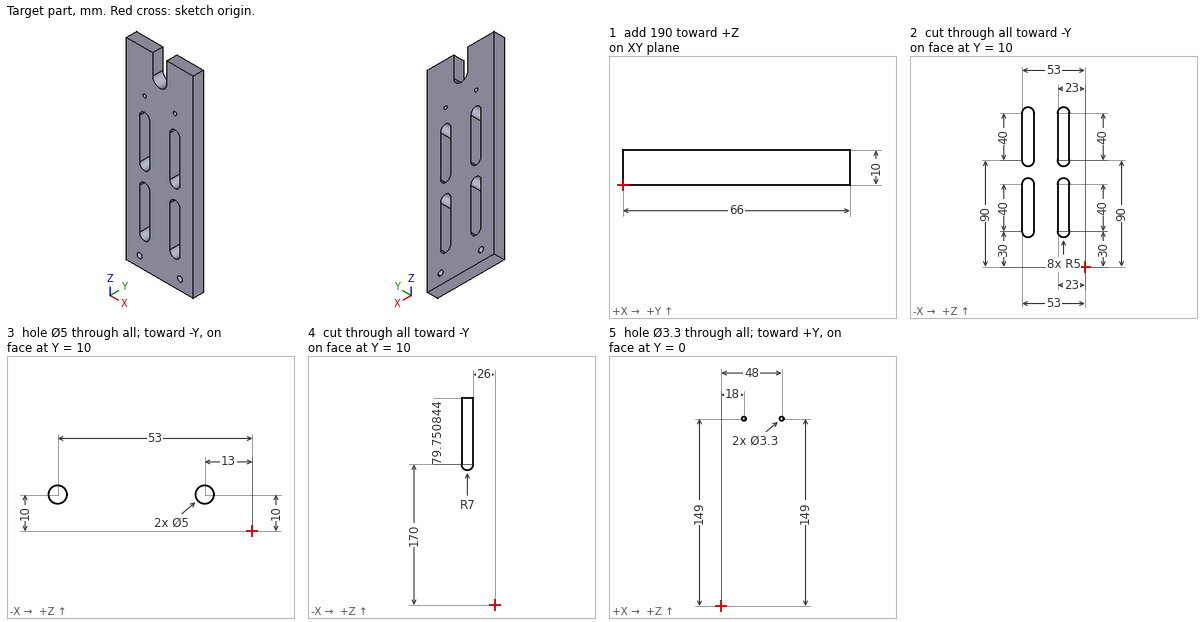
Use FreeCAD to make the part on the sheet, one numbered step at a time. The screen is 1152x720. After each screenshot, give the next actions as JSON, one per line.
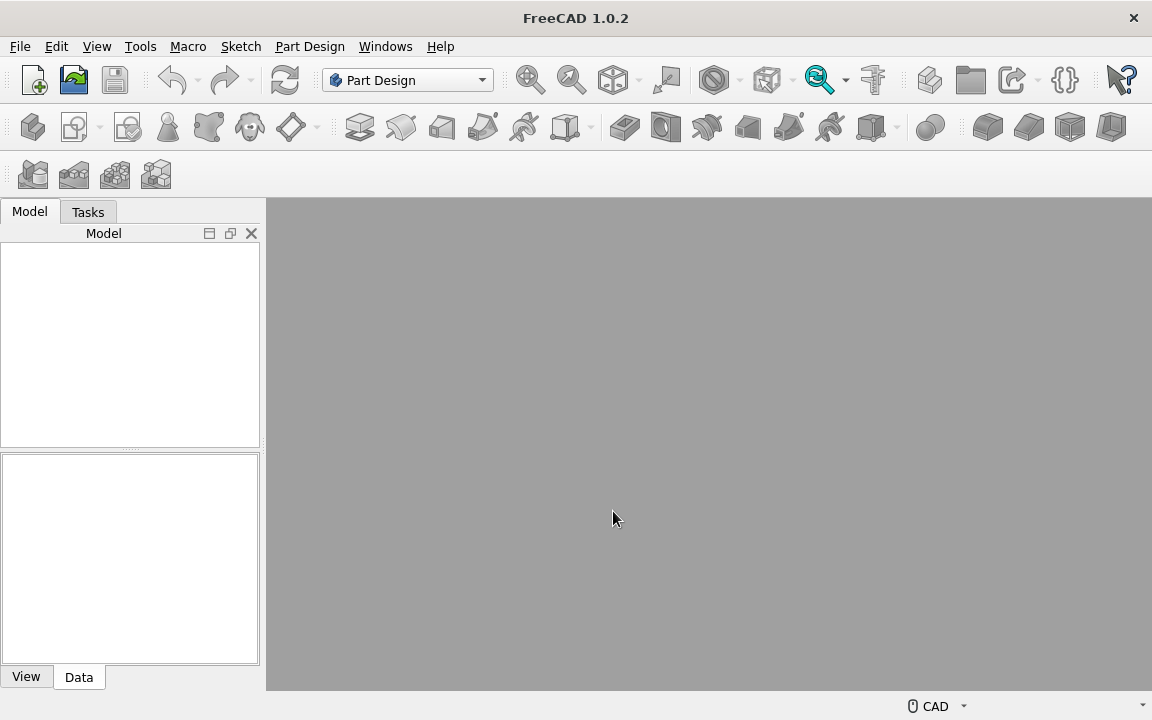
{"action": "left_click", "coordinate": [33, 80]}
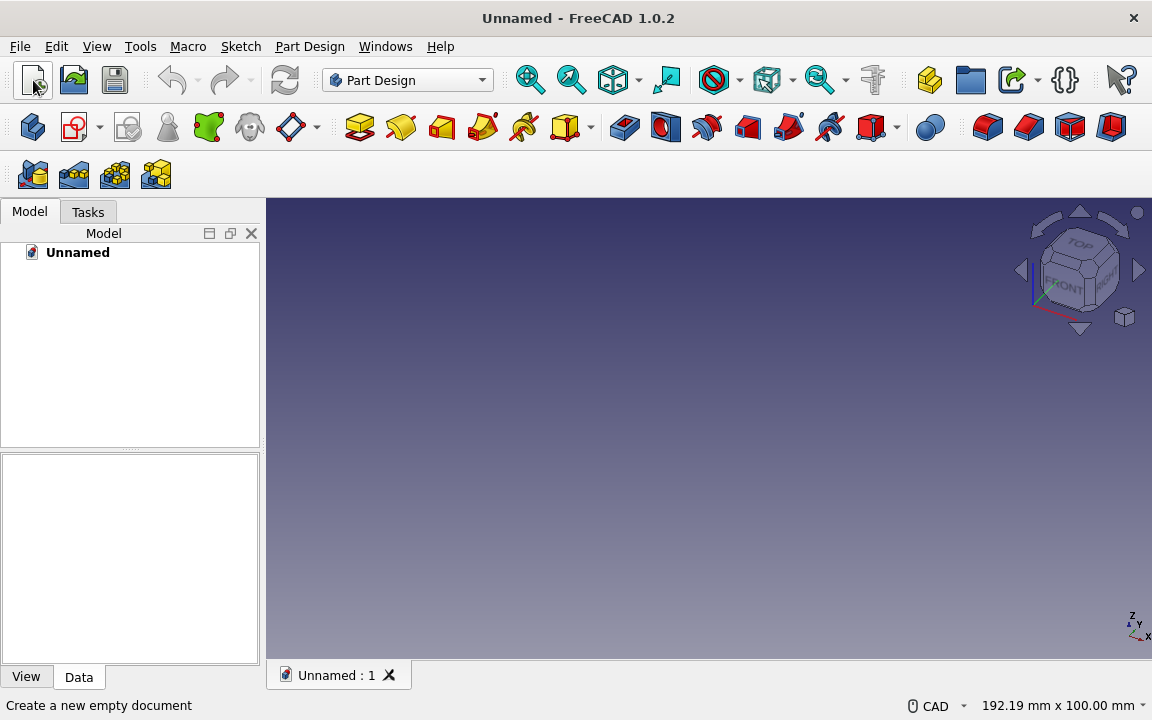
{"action": "left_click", "coordinate": [74, 128]}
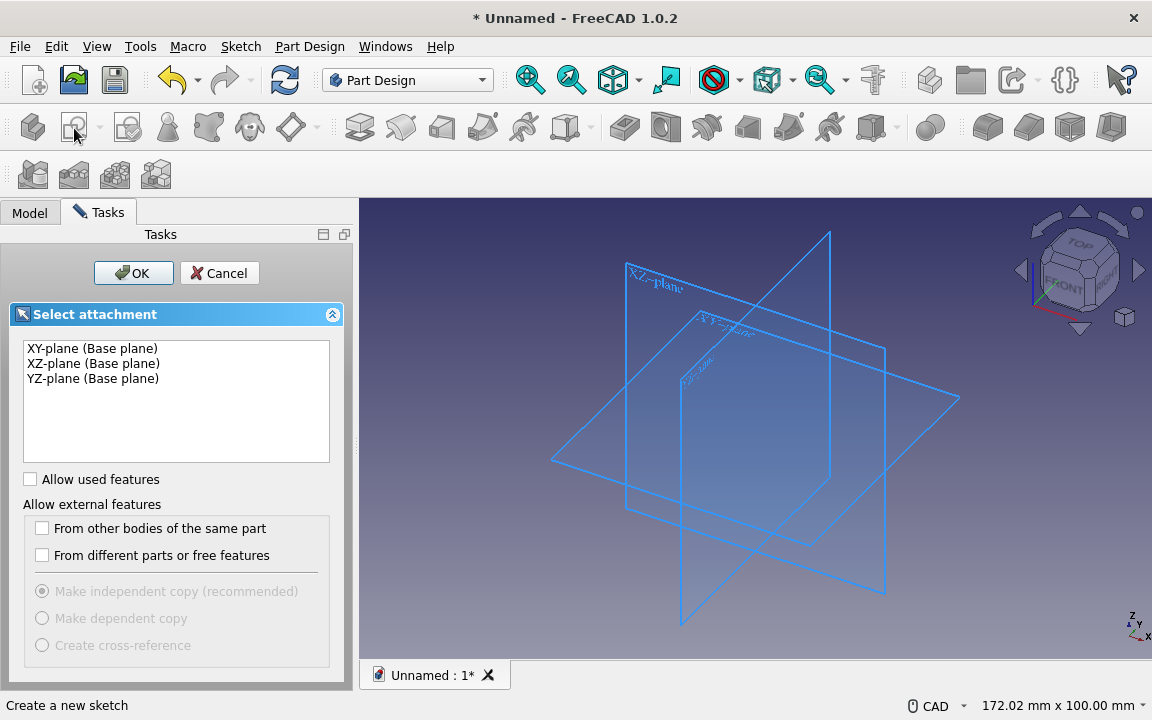
{"action": "left_click", "coordinate": [84, 348]}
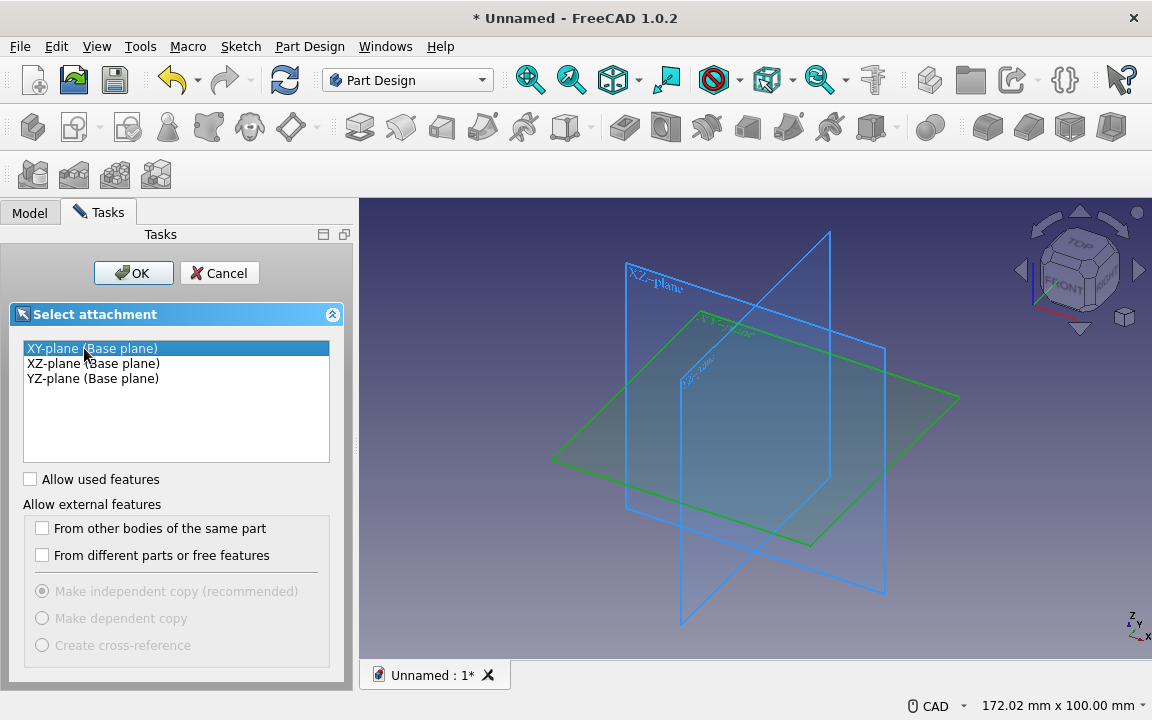
{"action": "left_click", "coordinate": [134, 273]}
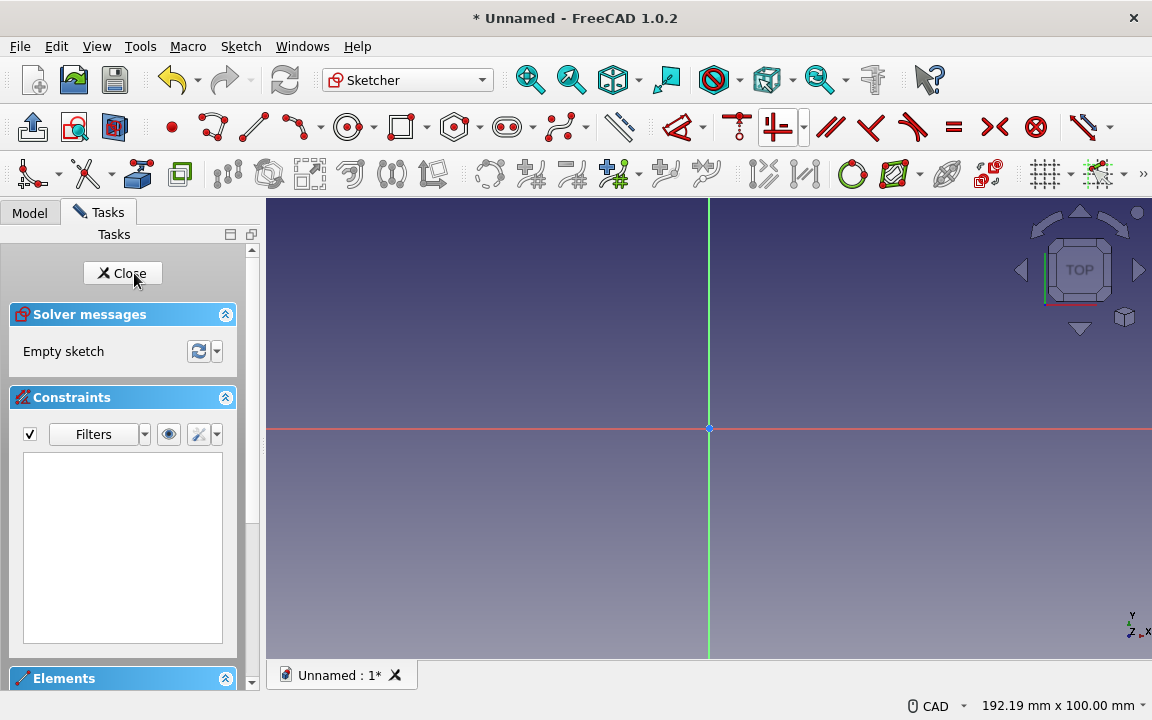
{"action": "scroll", "coordinate": [294, 533], "scroll_direction": "down", "scroll_amount": 1}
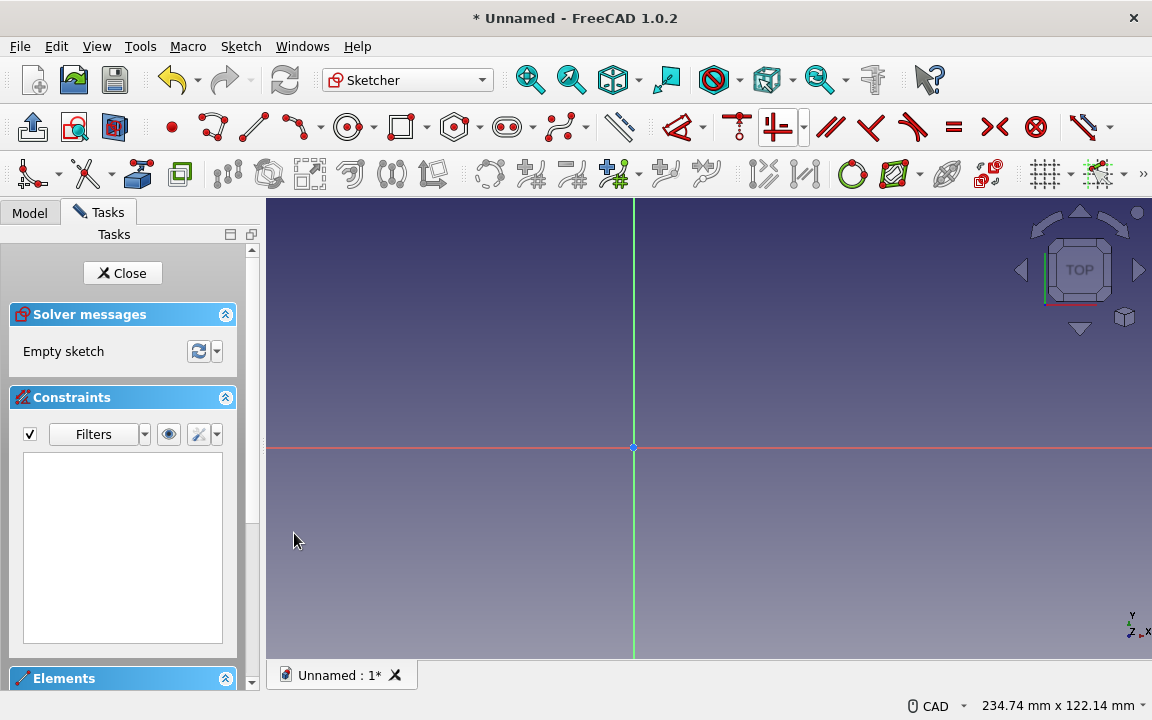
{"action": "scroll", "coordinate": [902, 429], "scroll_direction": "up", "scroll_amount": 3}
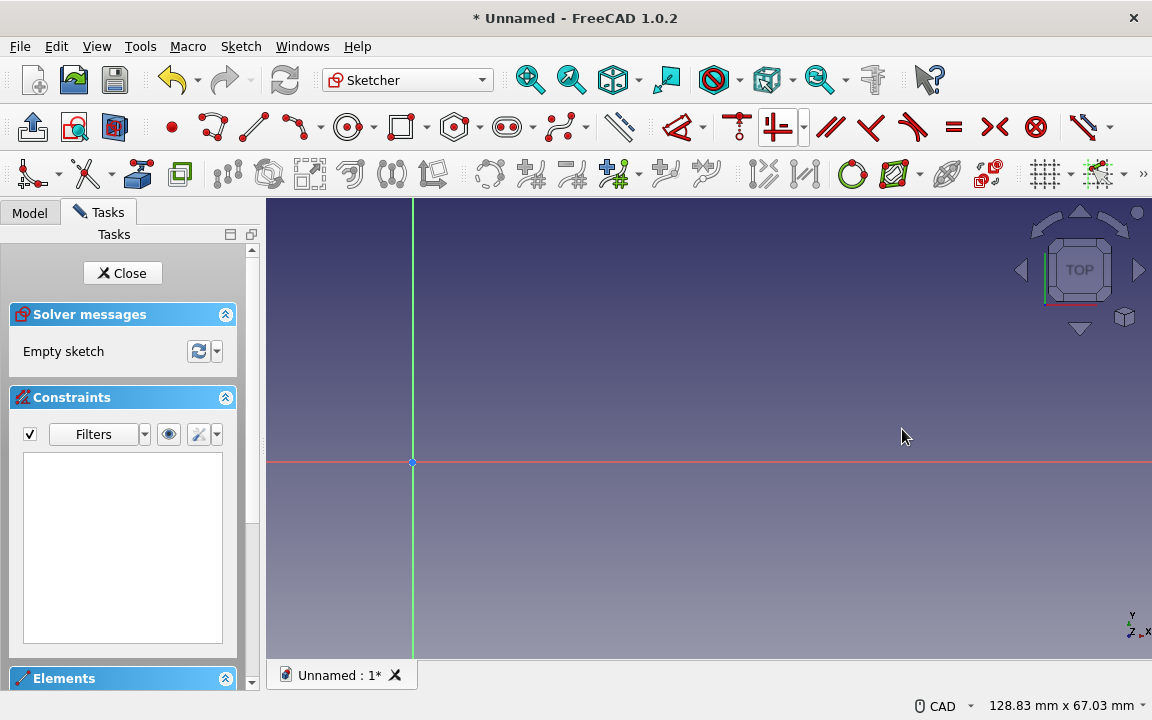
{"action": "left_click", "coordinate": [400, 128]}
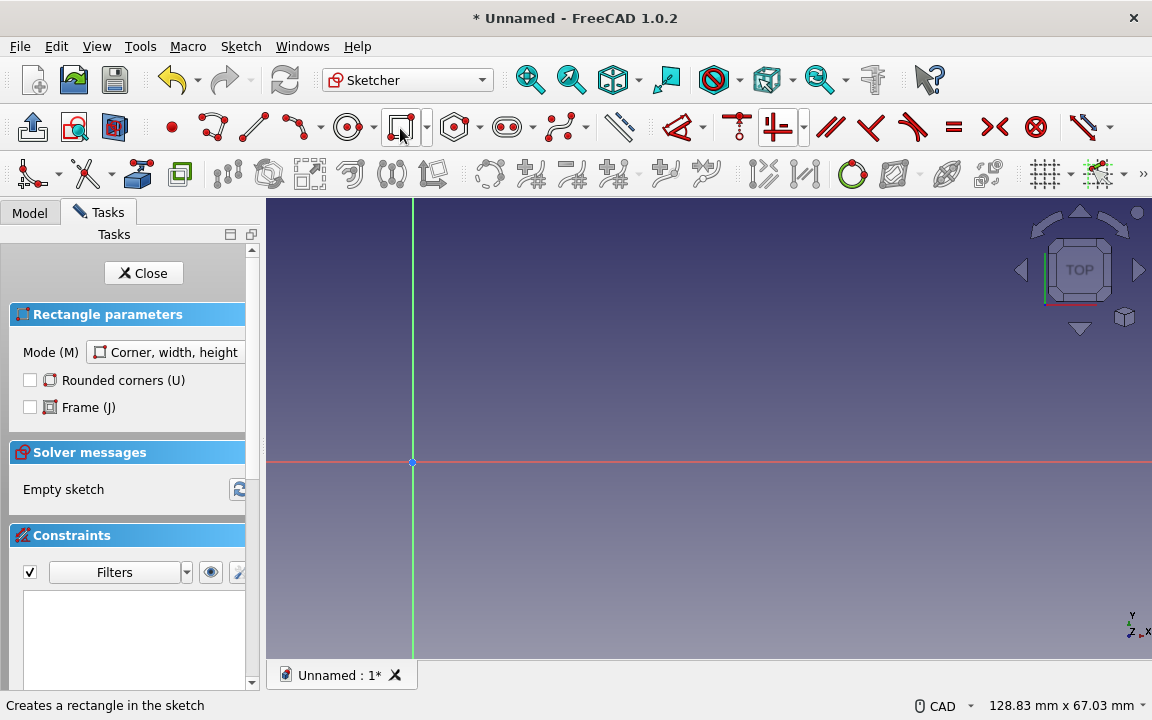
{"action": "left_click", "coordinate": [413, 462]}
{"action": "mouse_move", "coordinate": [867, 394]}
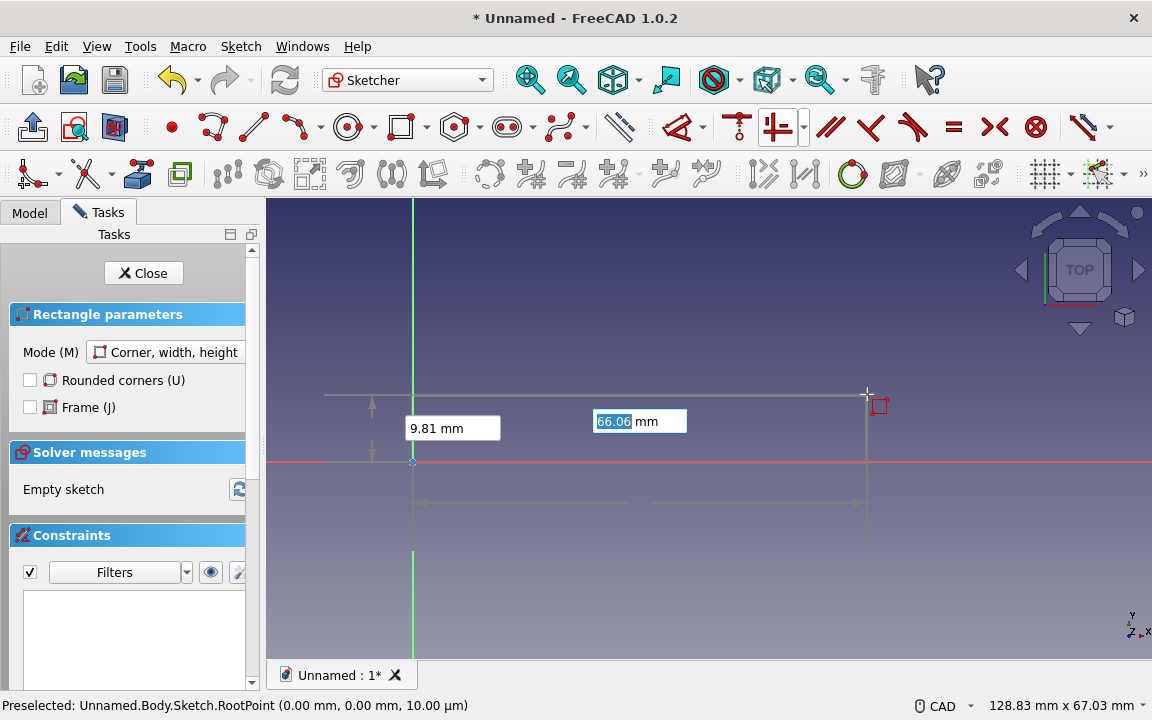
{"action": "type", "text": "66"}
{"action": "key", "text": "Tab"}
{"action": "type", "text": "10"}
{"action": "key", "text": "Return"}
{"action": "key", "text": "Escape"}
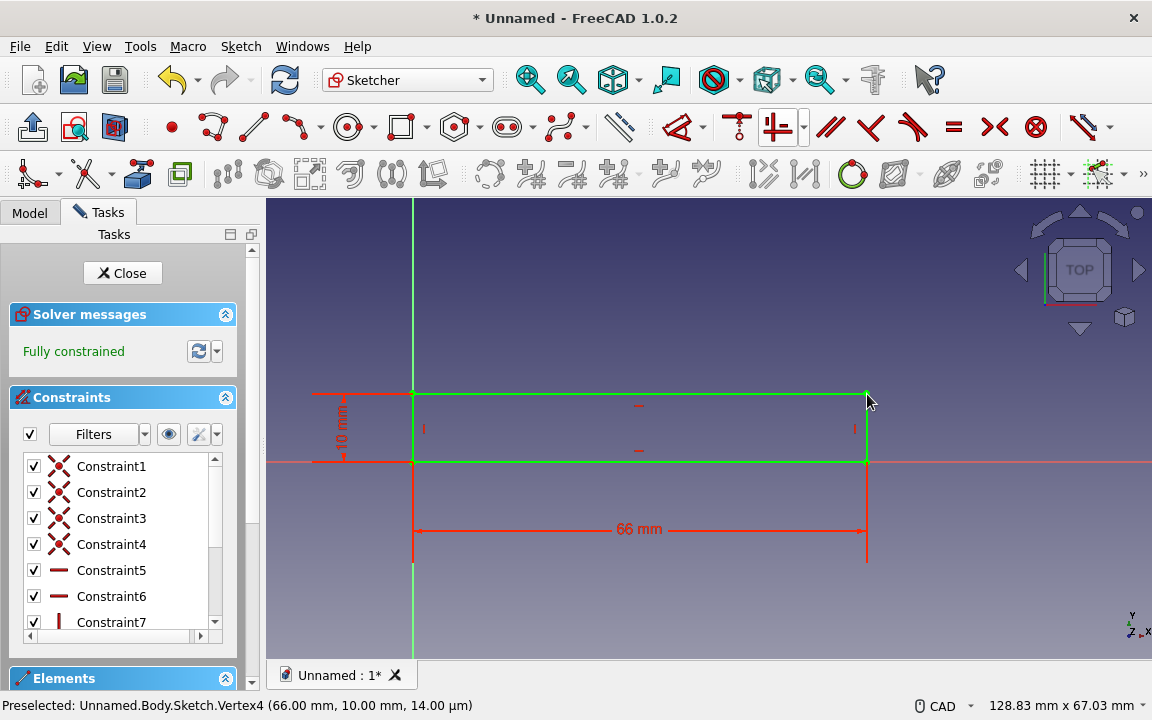
{"action": "left_click", "coordinate": [123, 273]}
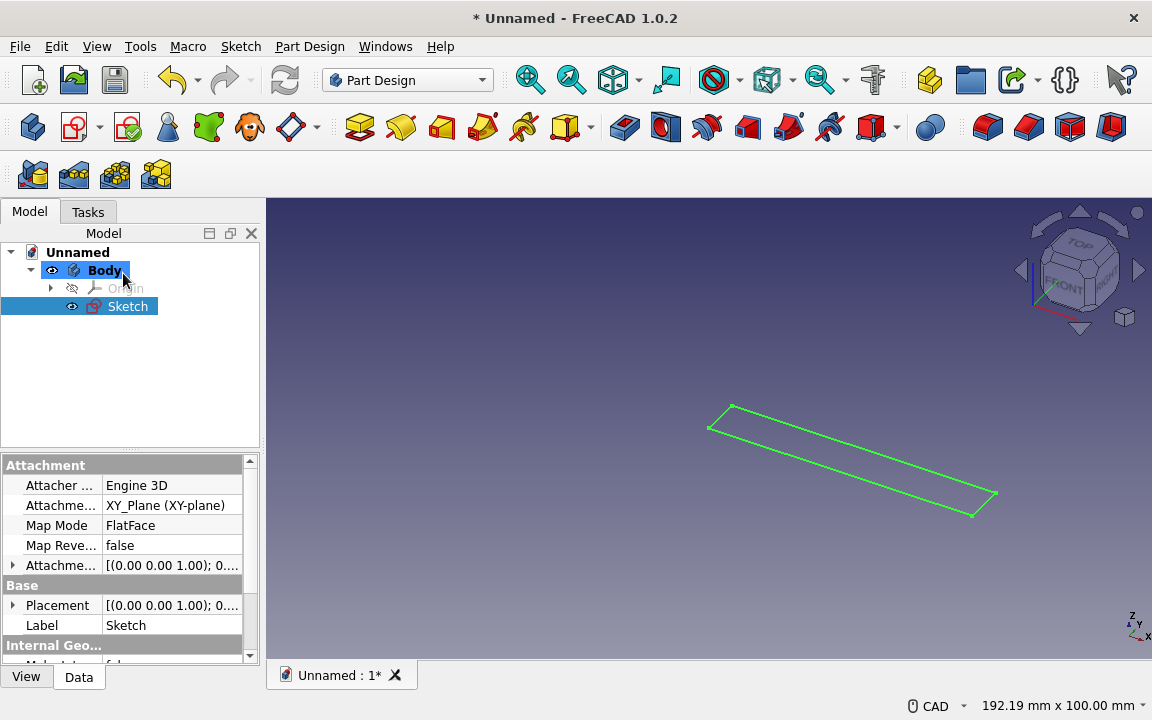
{"action": "left_click", "coordinate": [360, 128]}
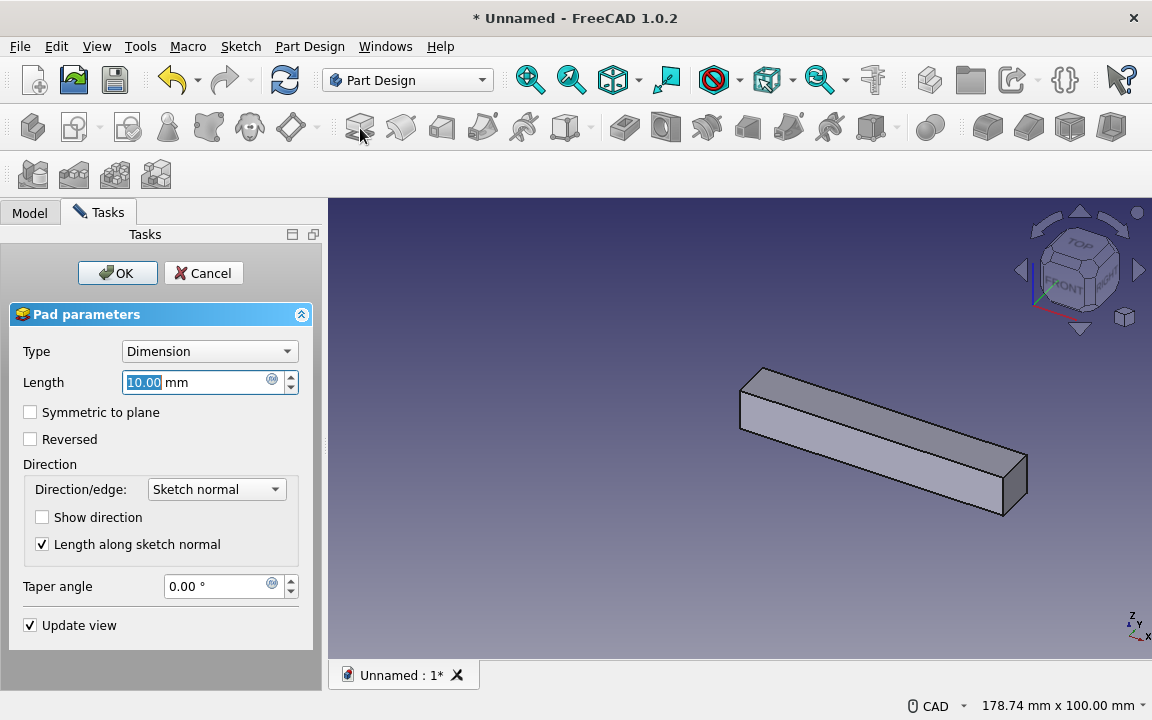
{"action": "type", "text": "190"}
{"action": "key", "text": "Tab"}